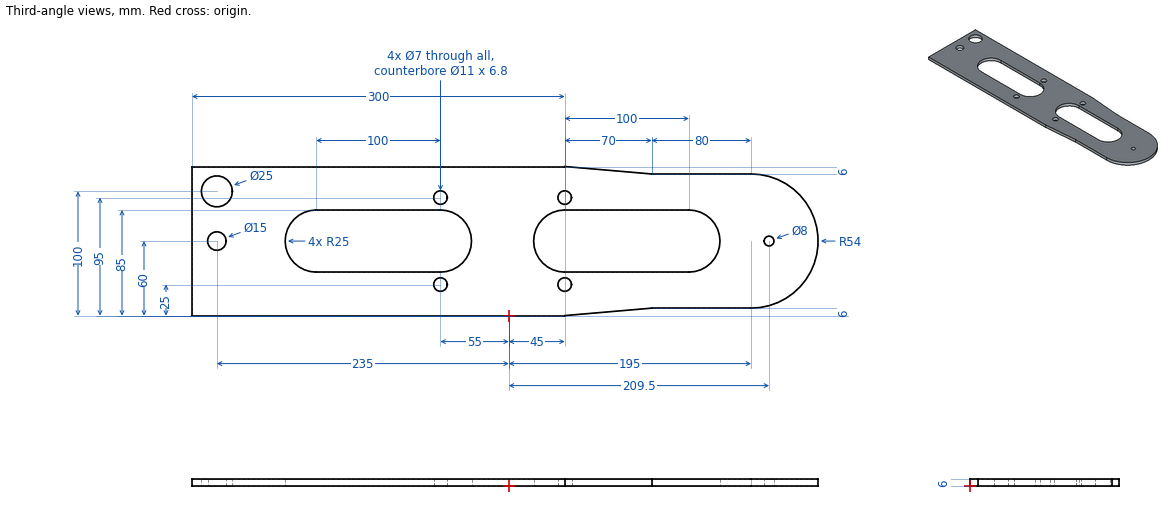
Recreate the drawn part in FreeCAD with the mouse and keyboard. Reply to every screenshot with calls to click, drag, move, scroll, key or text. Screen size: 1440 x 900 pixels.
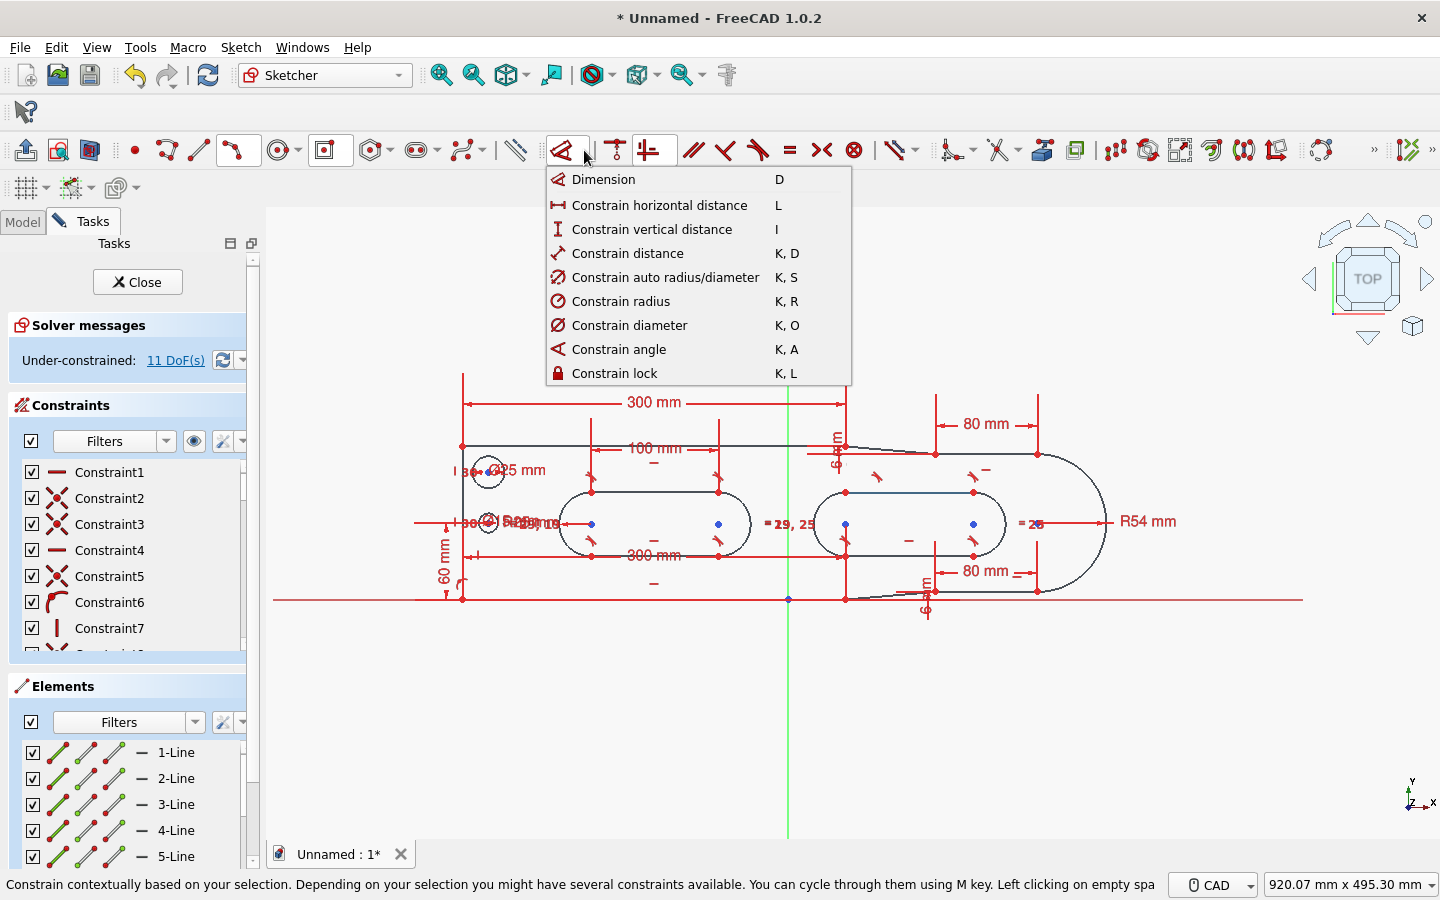
click(699, 205)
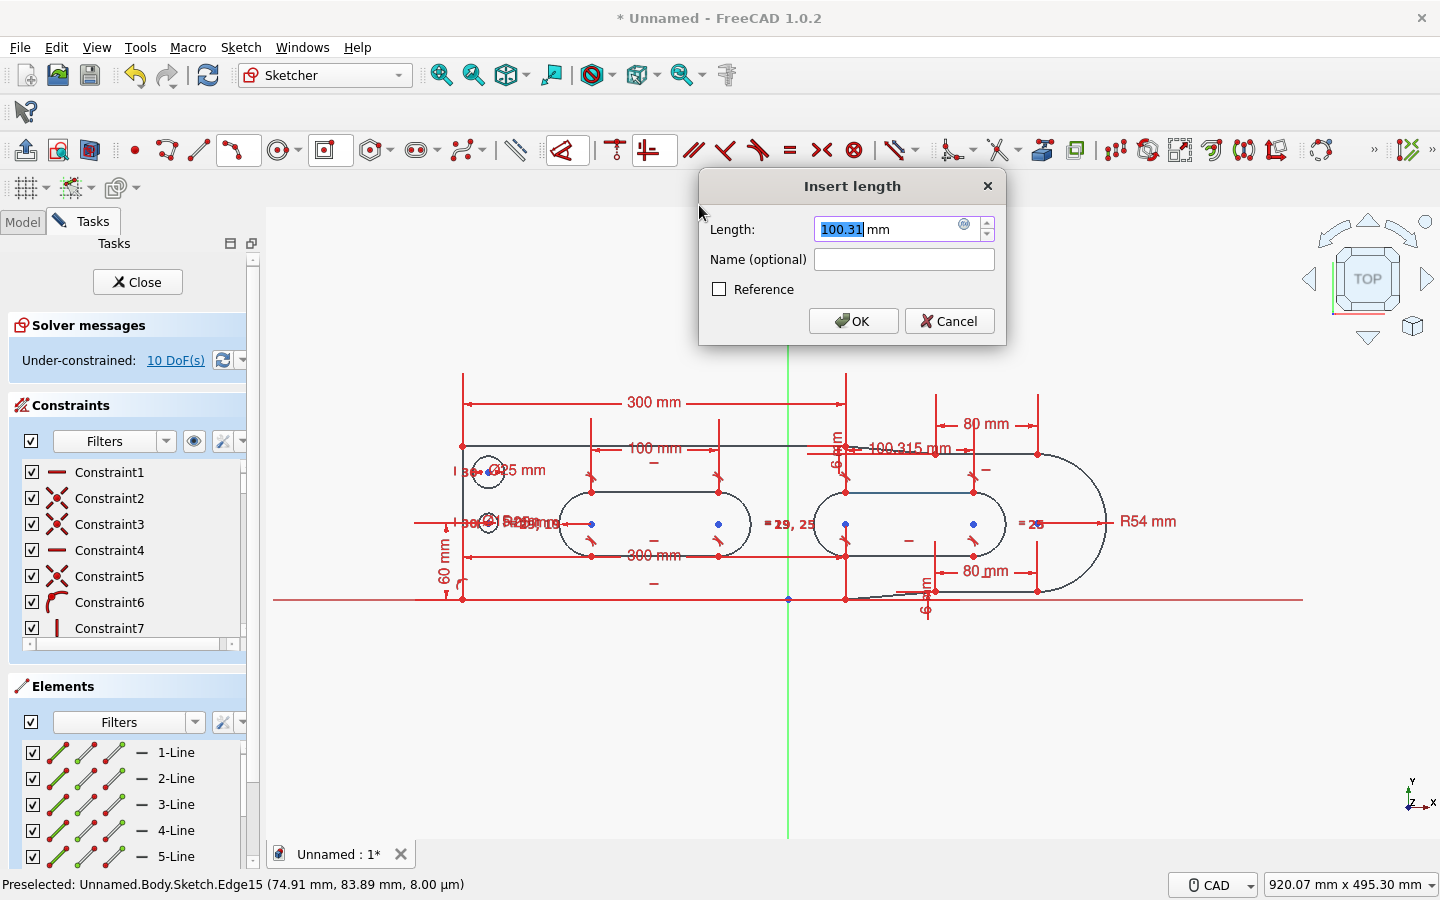
text(100)
key(Return)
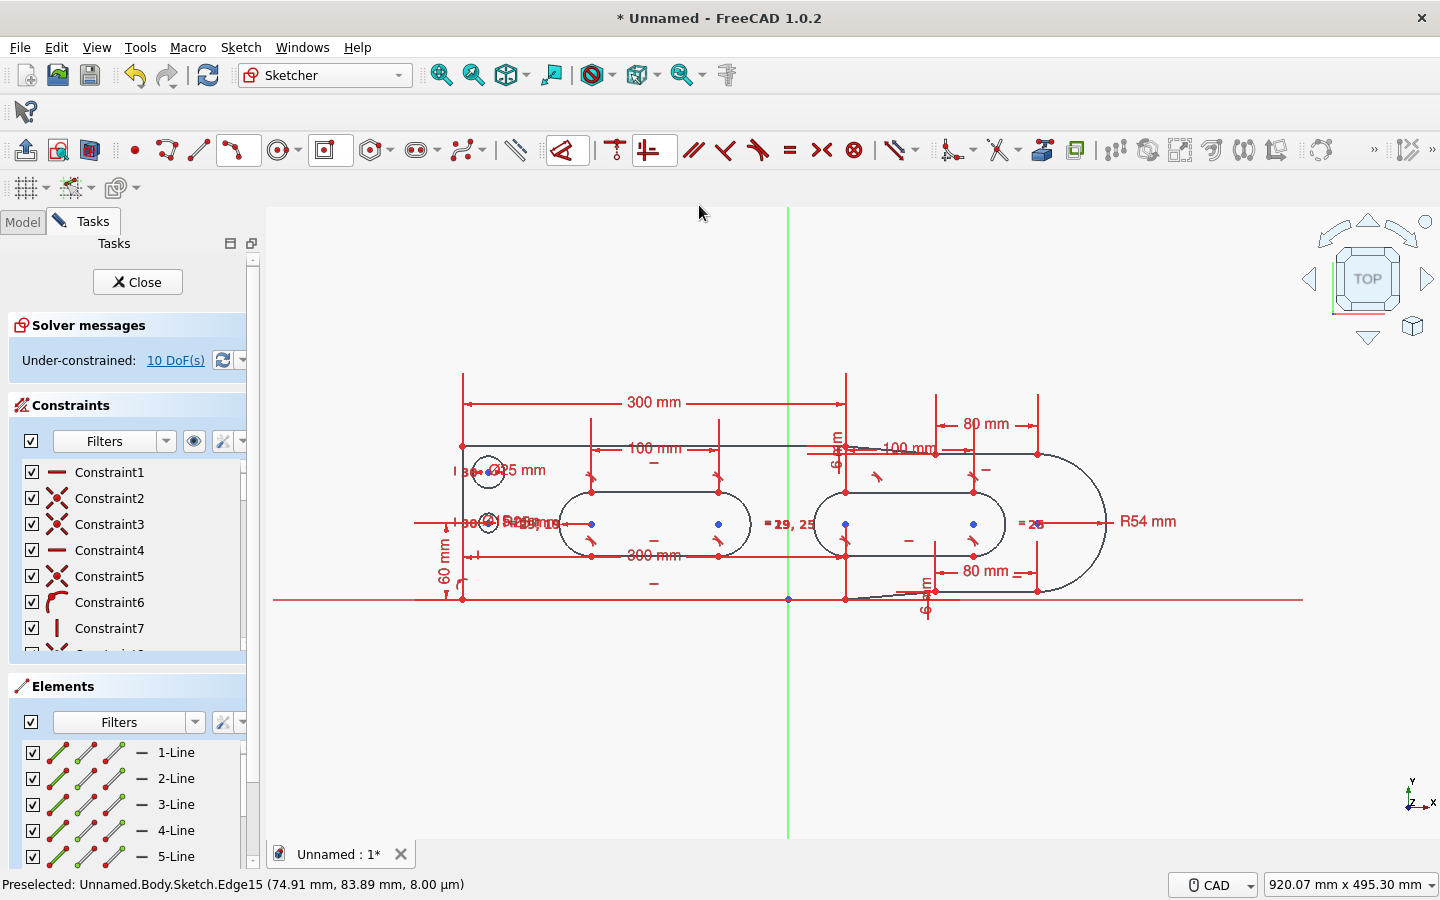
click(846, 446)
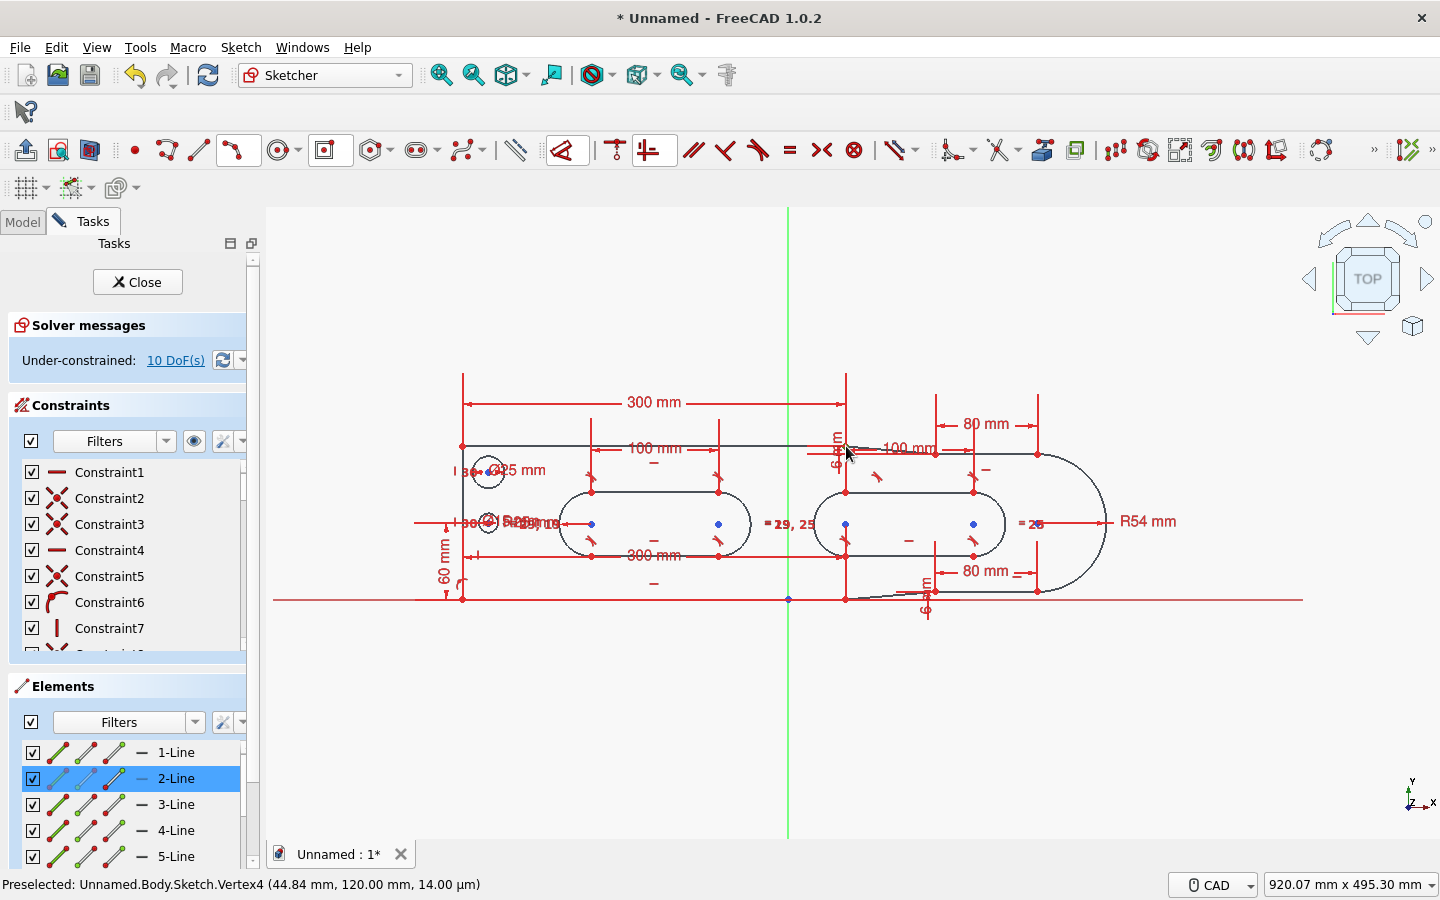
click(584, 150)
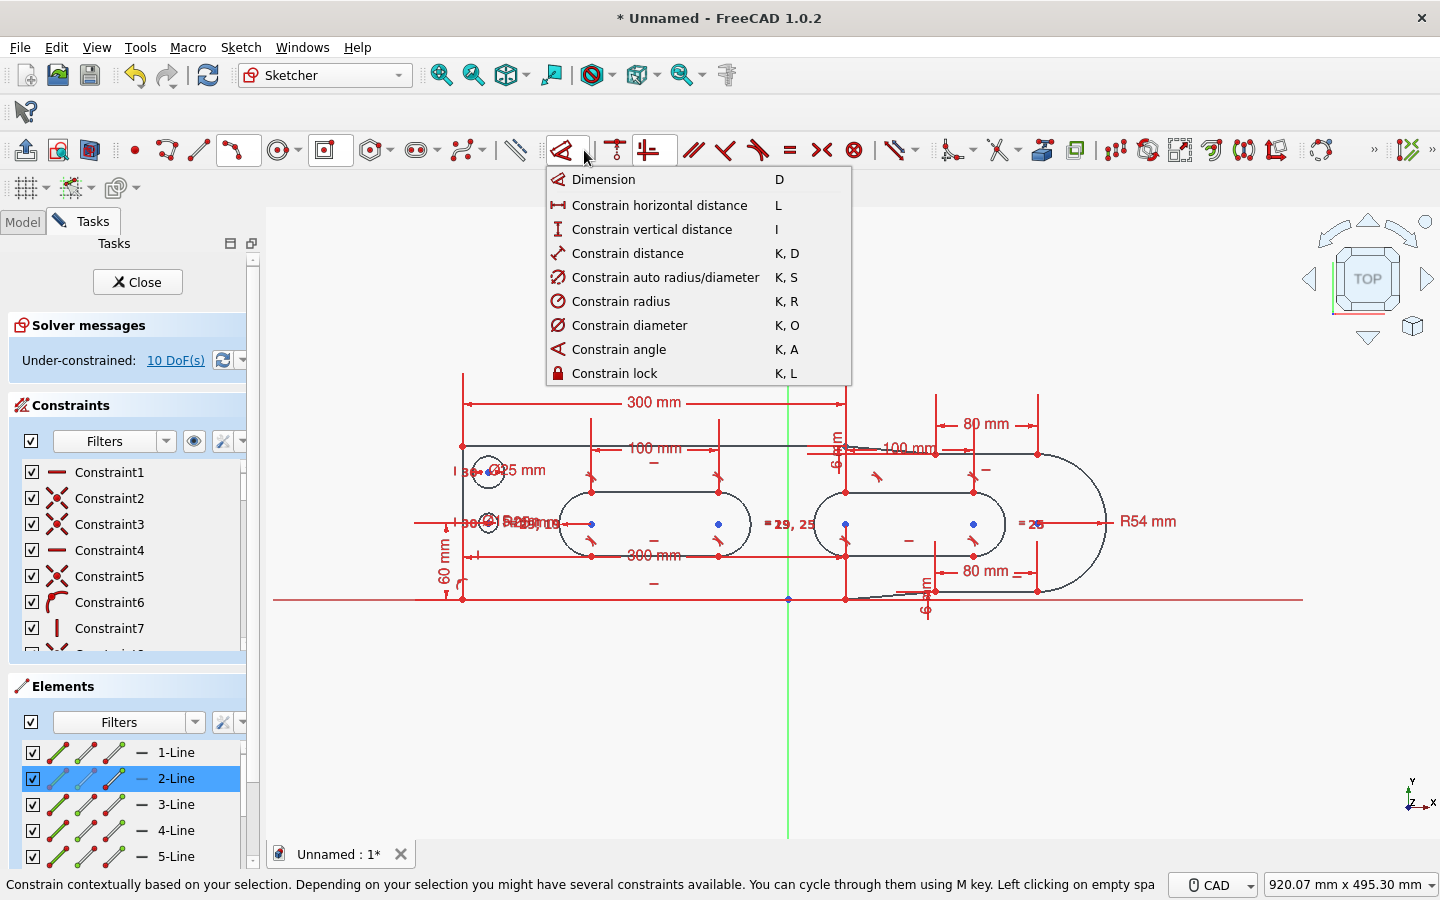
click(699, 205)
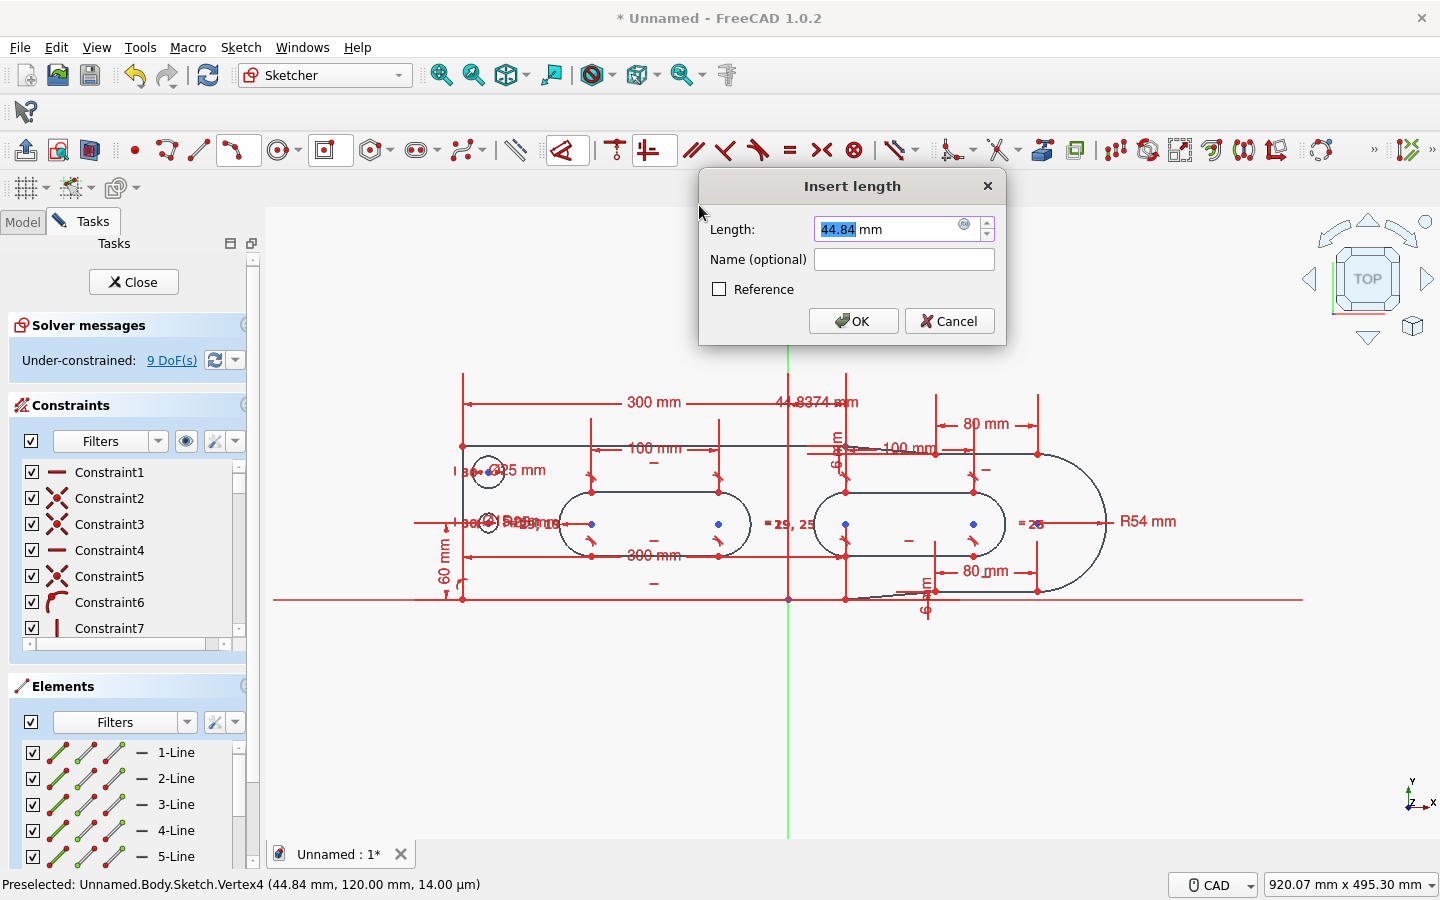
text(45)
key(Return)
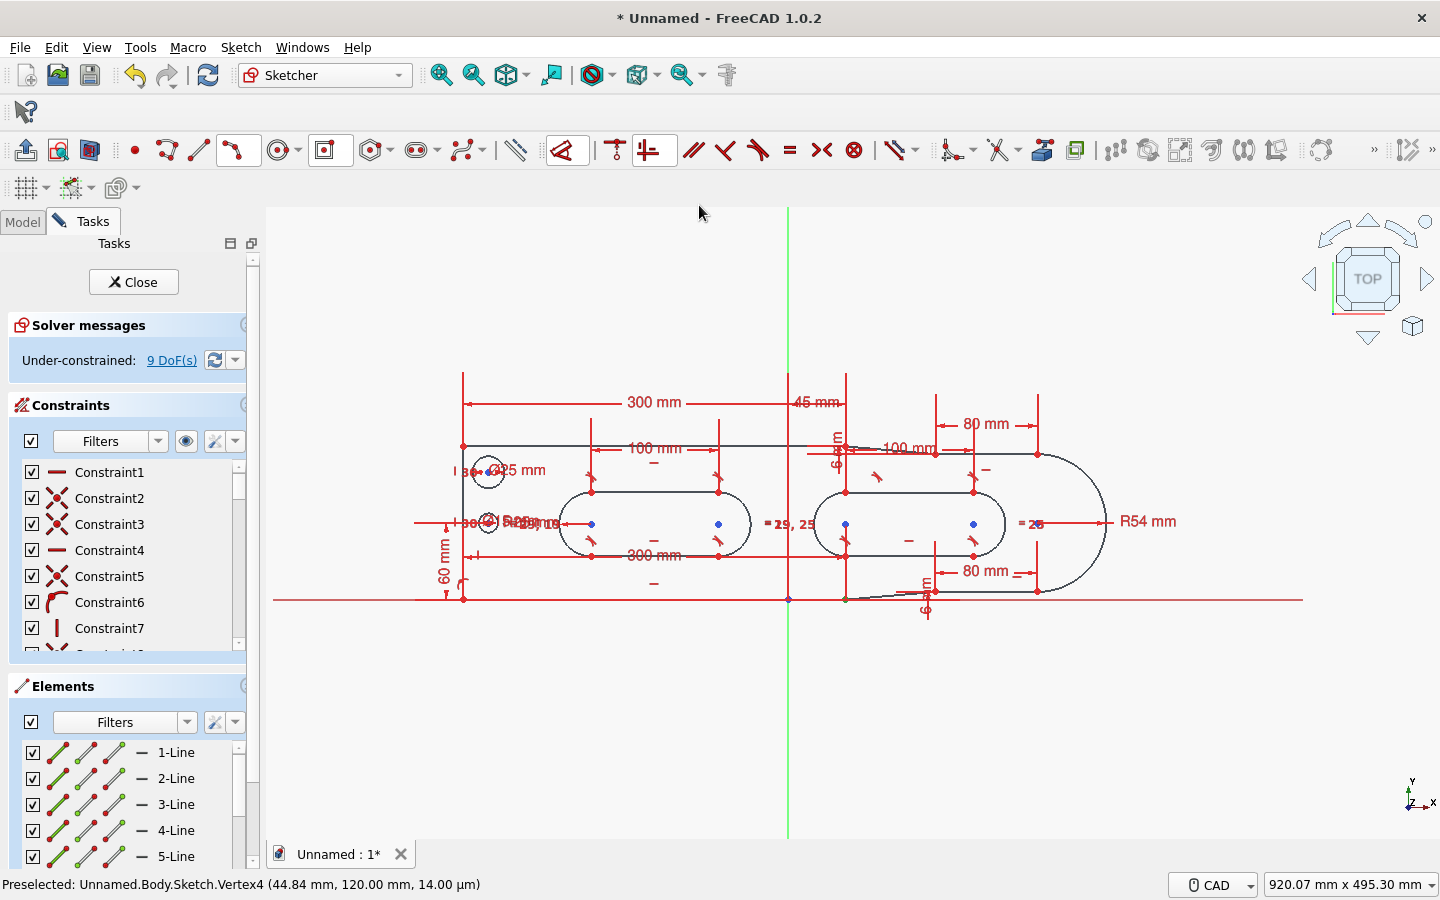
click(591, 492)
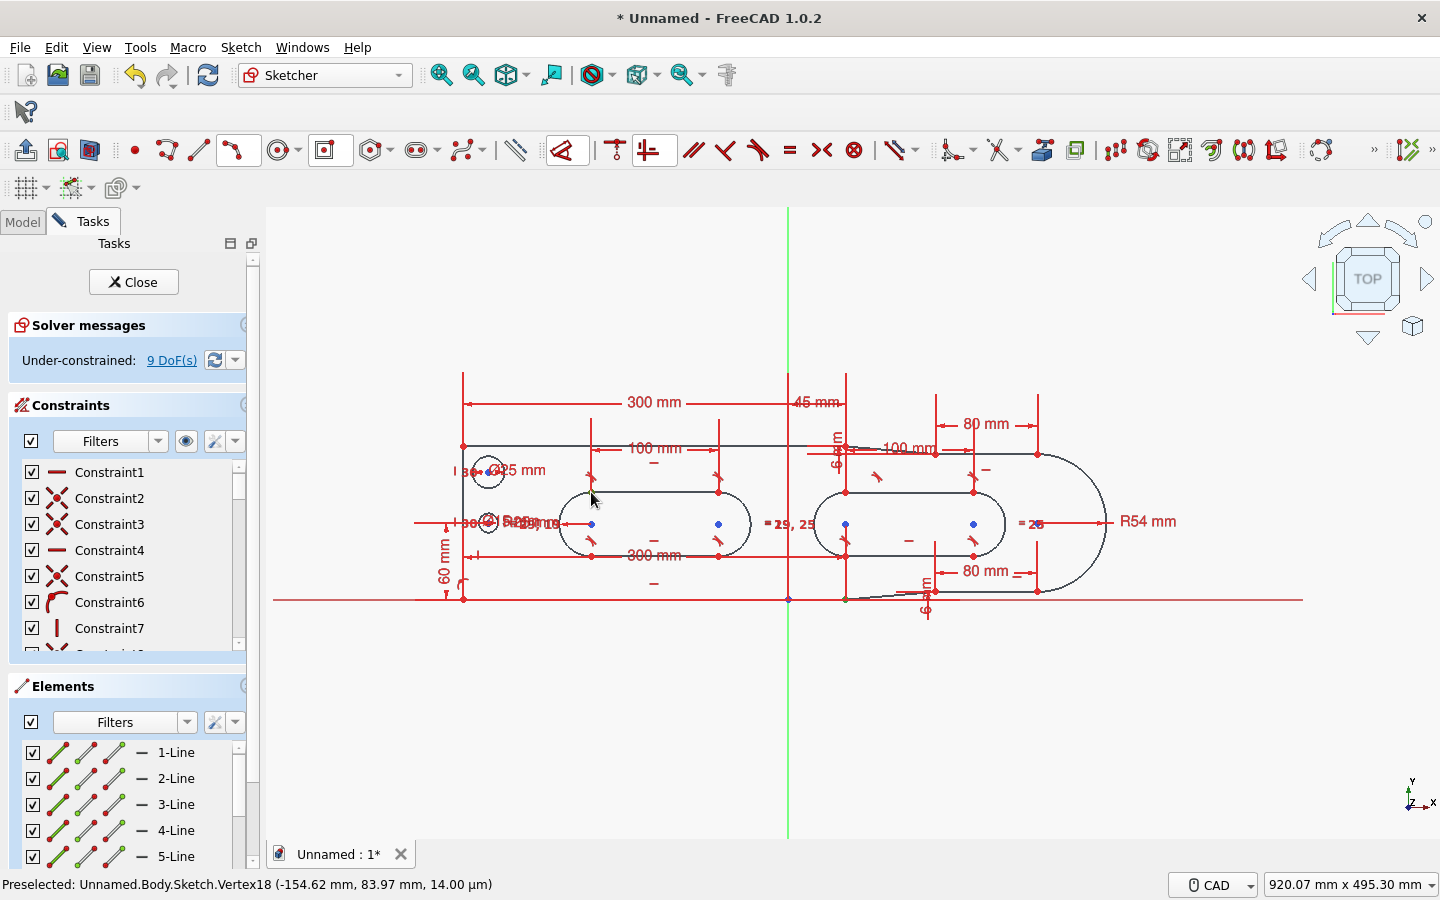
key(i)